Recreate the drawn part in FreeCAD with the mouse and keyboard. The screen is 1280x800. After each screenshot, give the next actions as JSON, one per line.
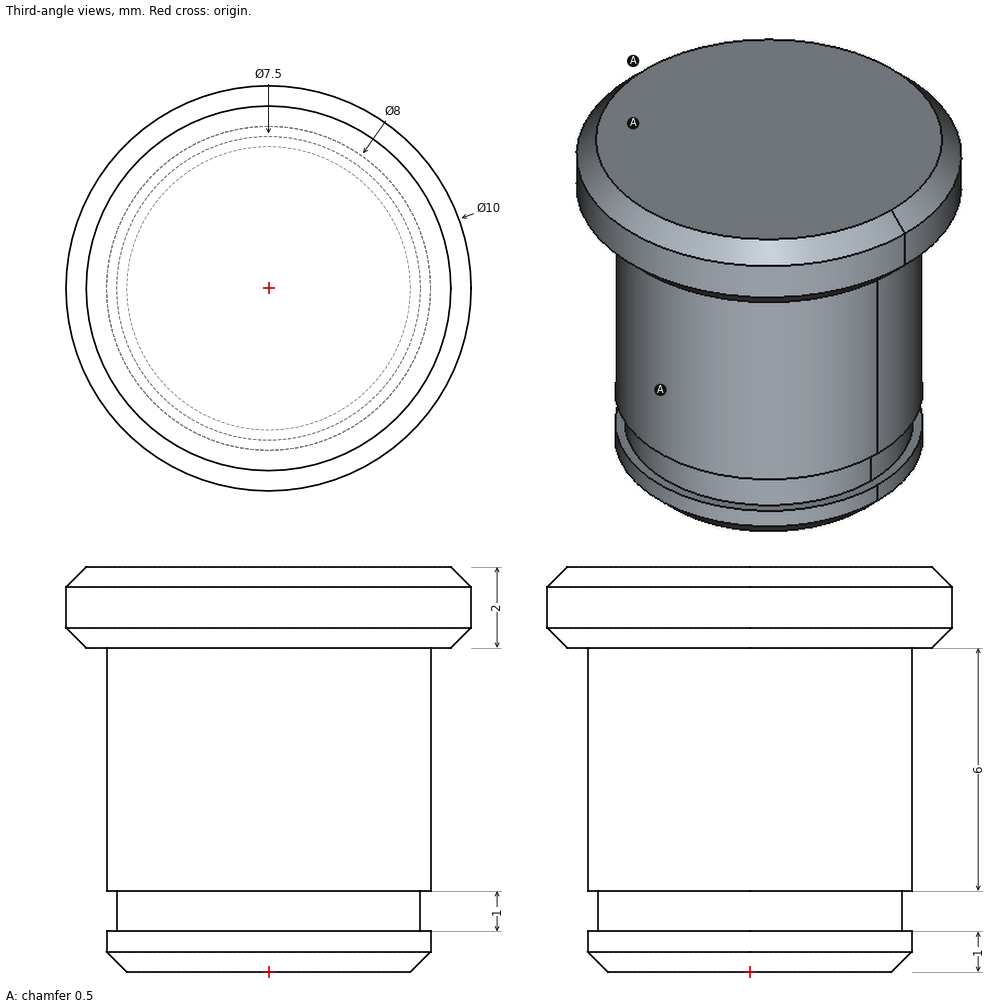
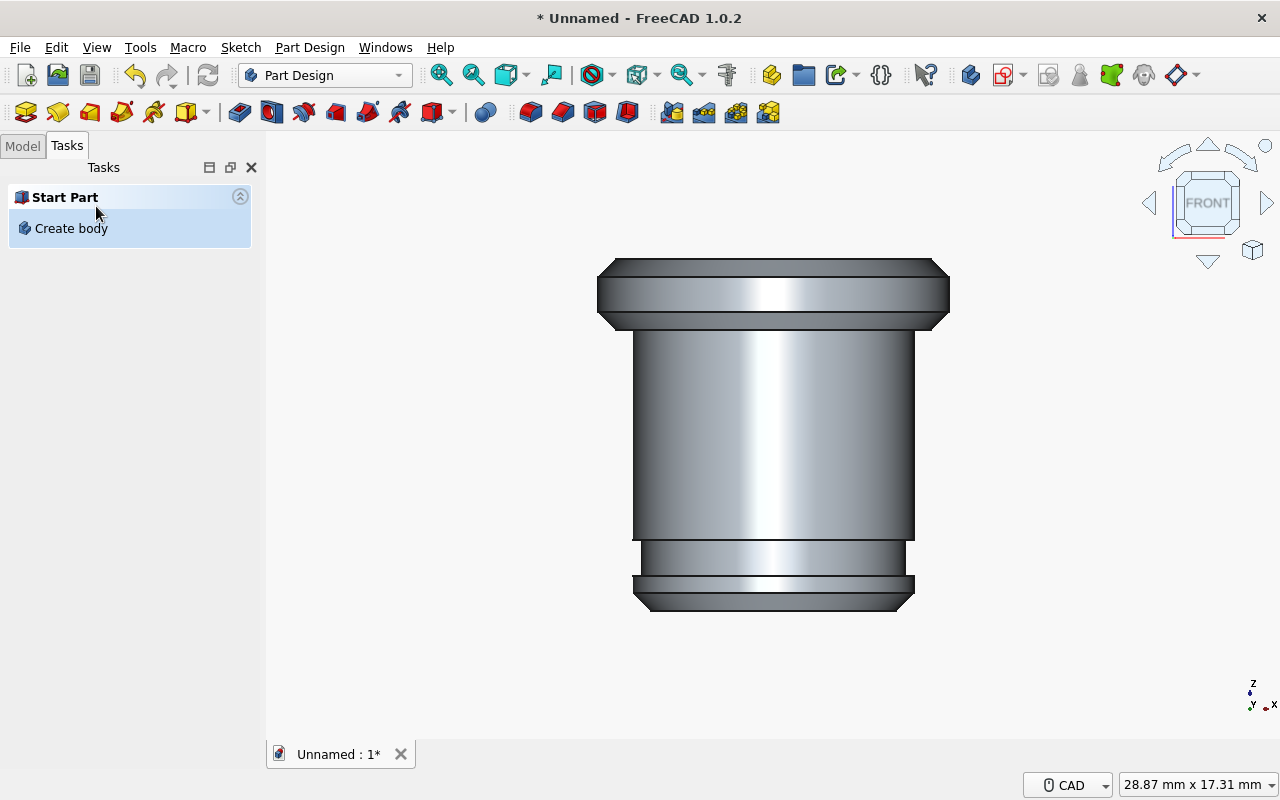
{"action": "key", "text": "0"}